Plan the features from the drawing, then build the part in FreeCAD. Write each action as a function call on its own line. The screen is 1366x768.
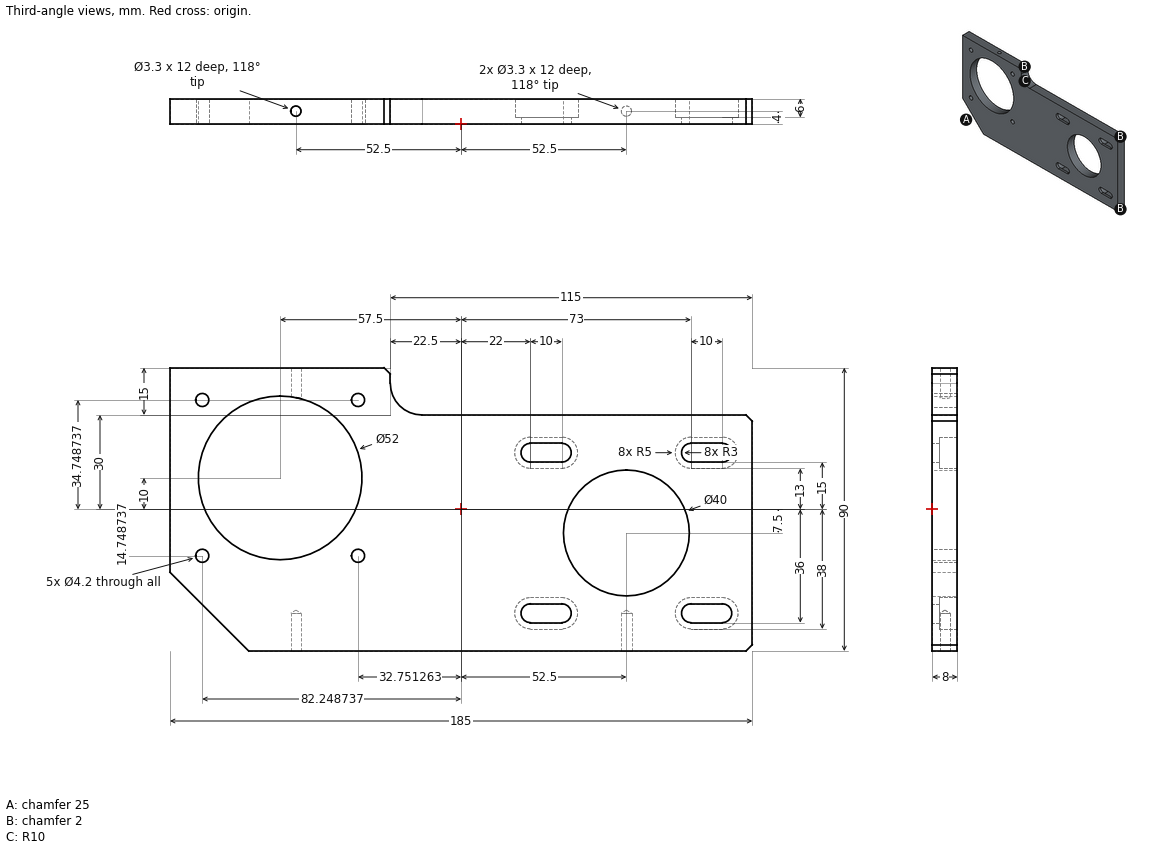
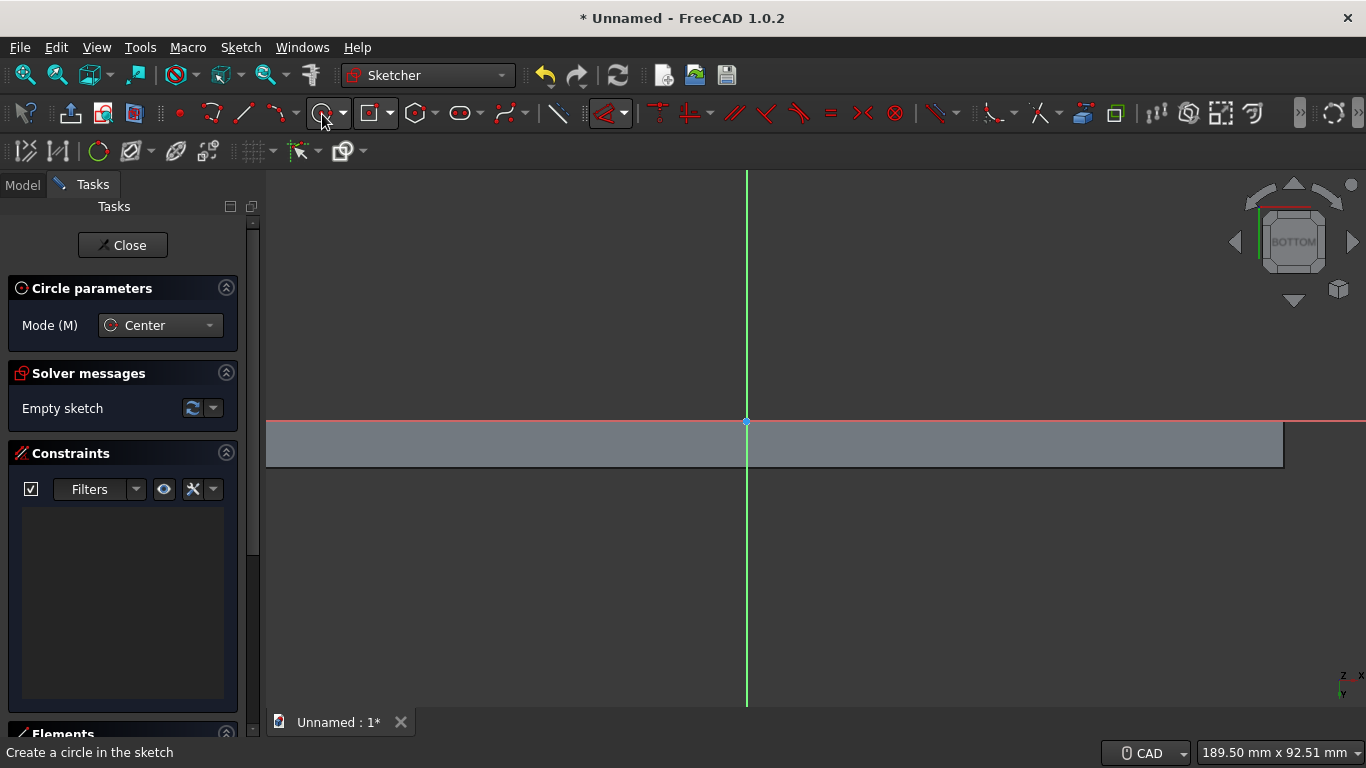
scroll(1051, 445, up, 5)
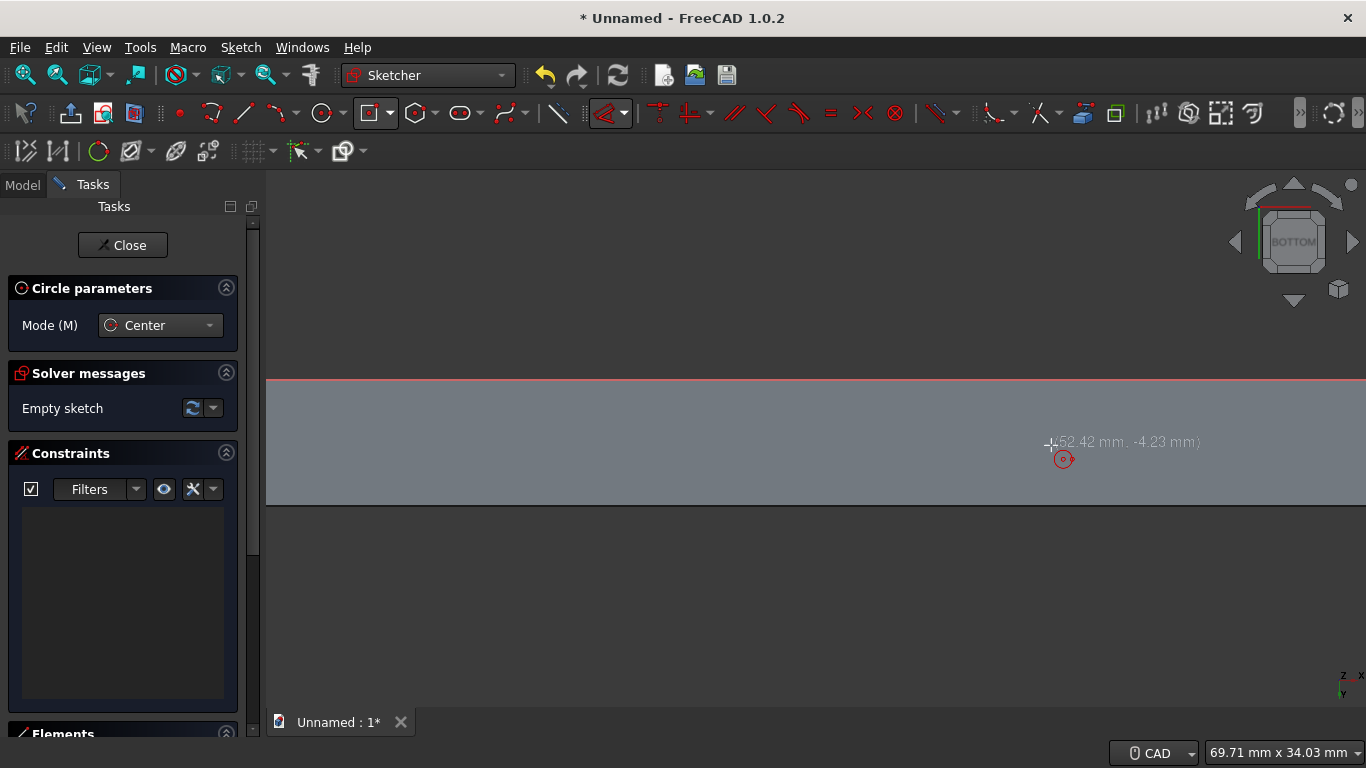
click(1051, 443)
click(1069, 425)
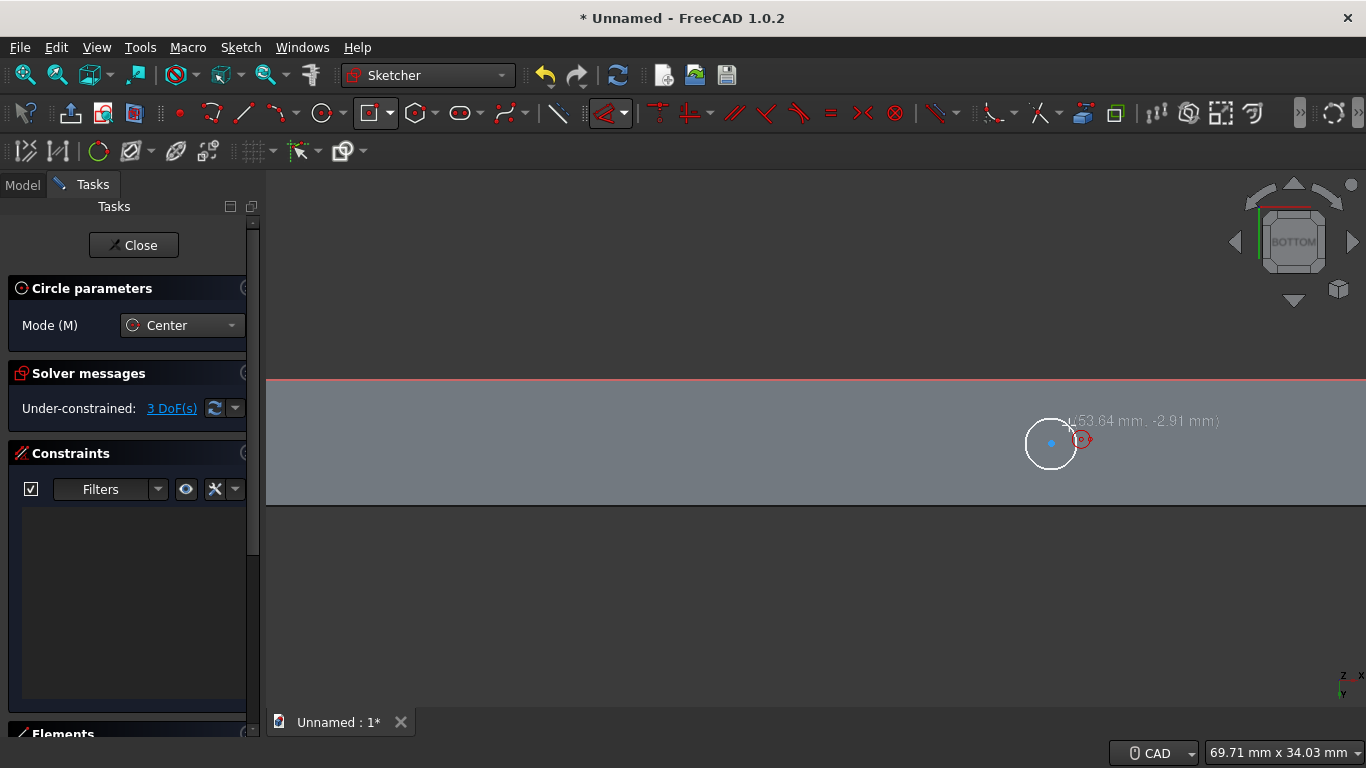
scroll(1053, 447, down, 5)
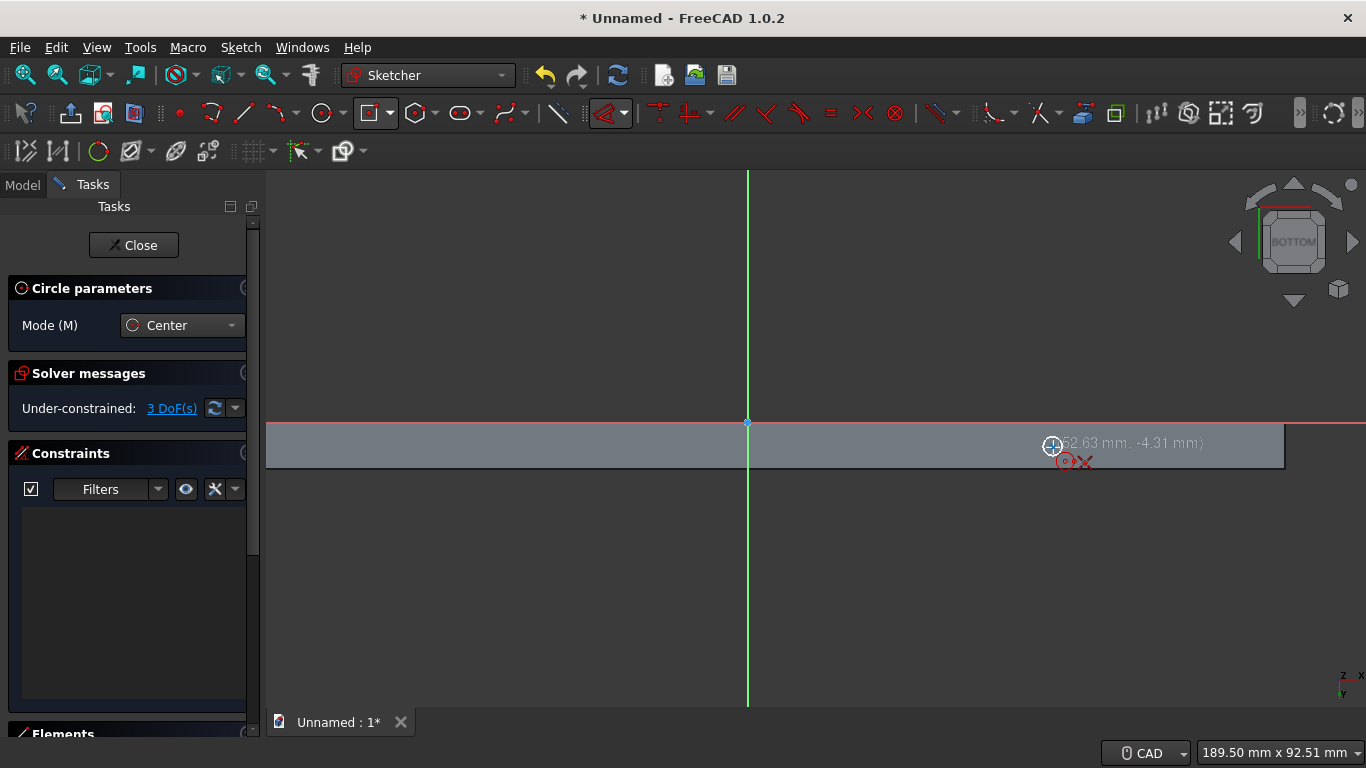
scroll(443, 446, up, 5)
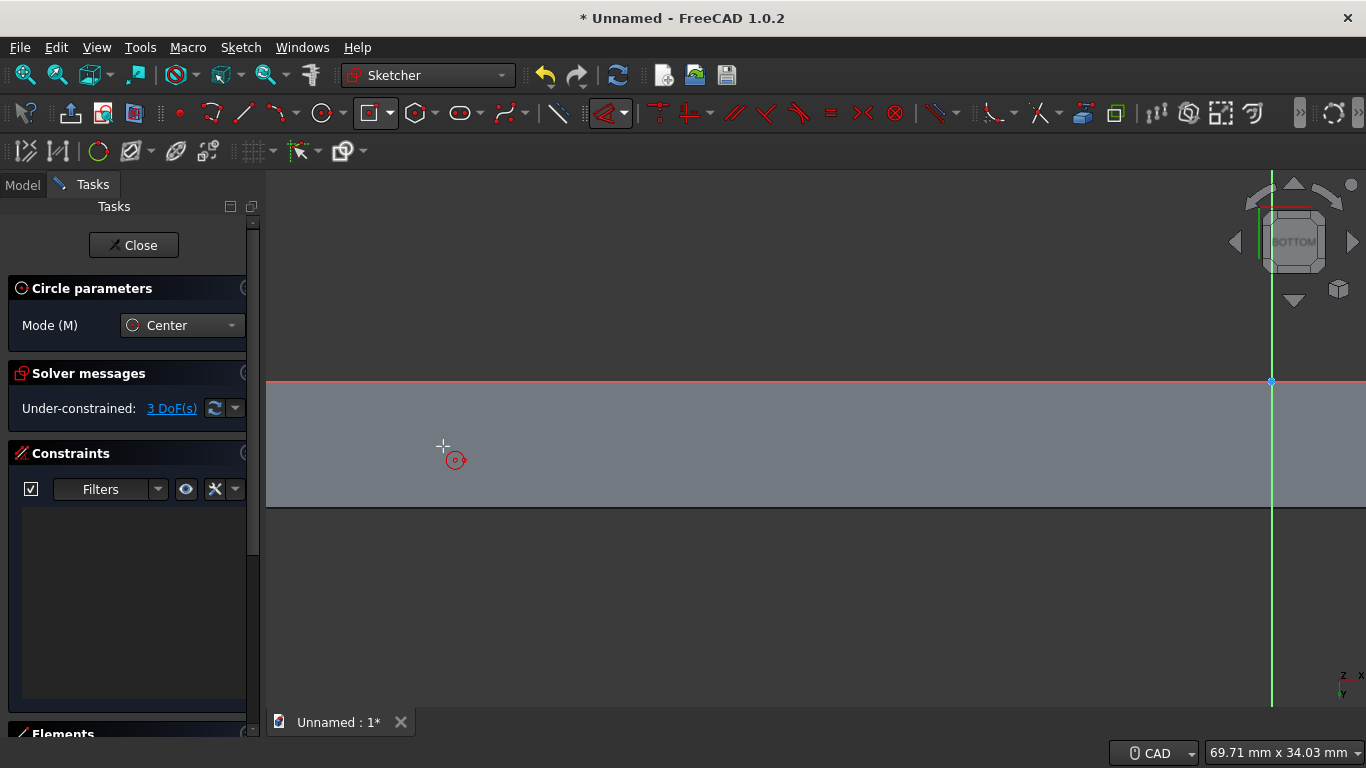
click(443, 445)
click(462, 426)
key(Escape)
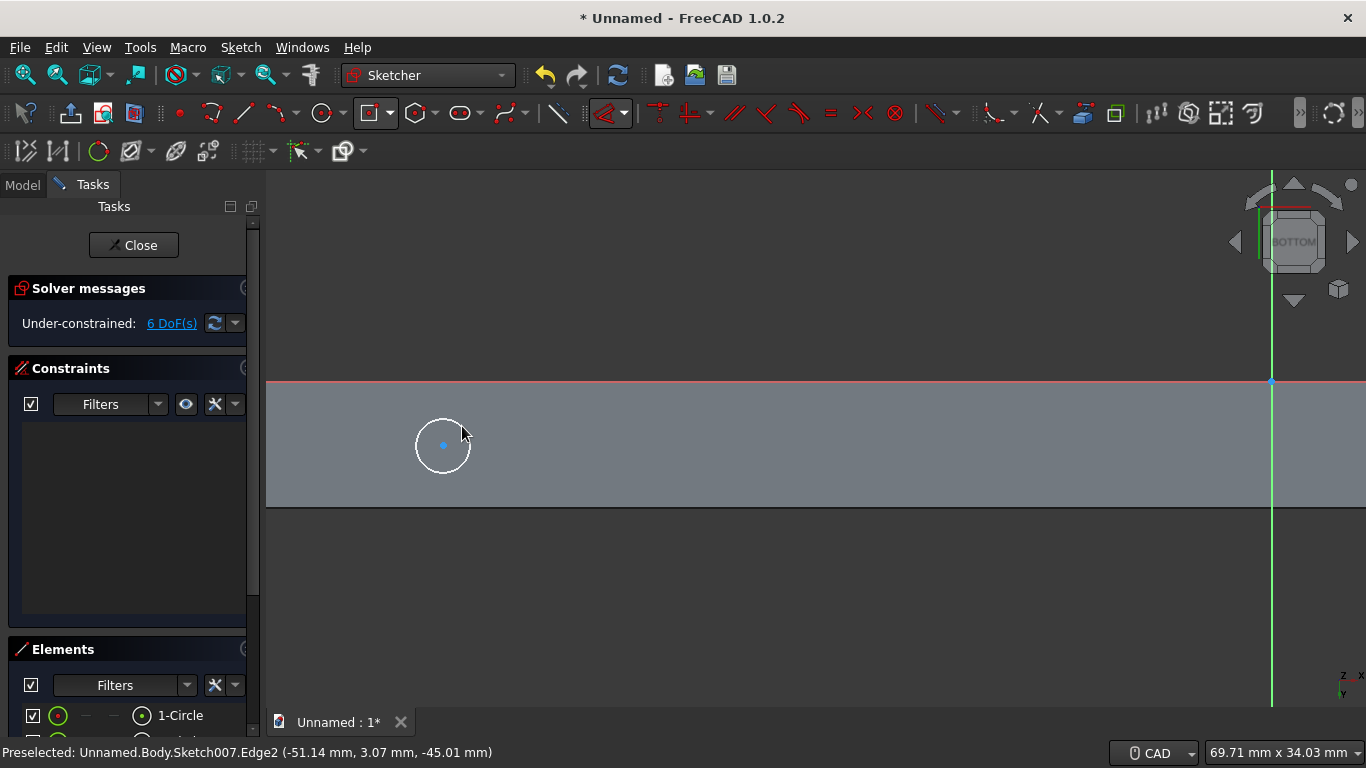
scroll(442, 446, down, 5)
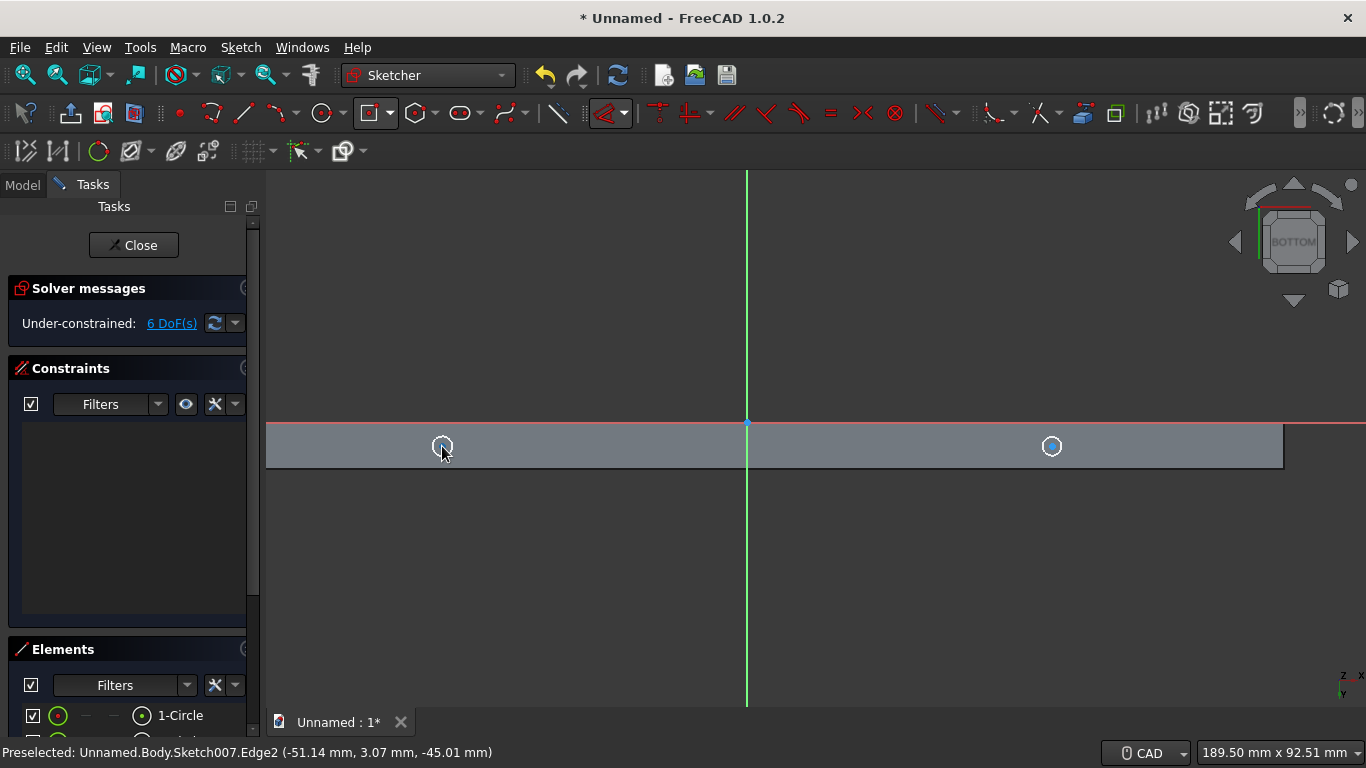
scroll(1059, 440, up, 2)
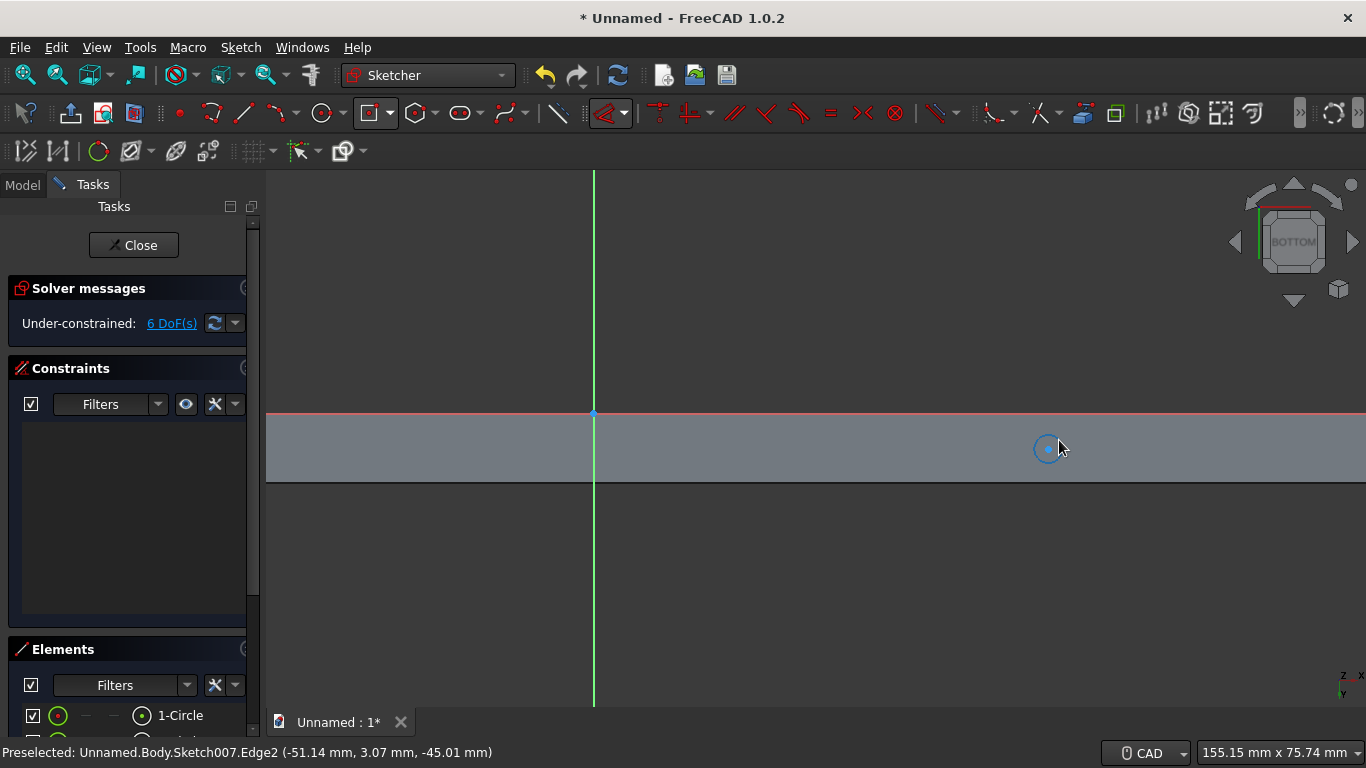
click(1058, 439)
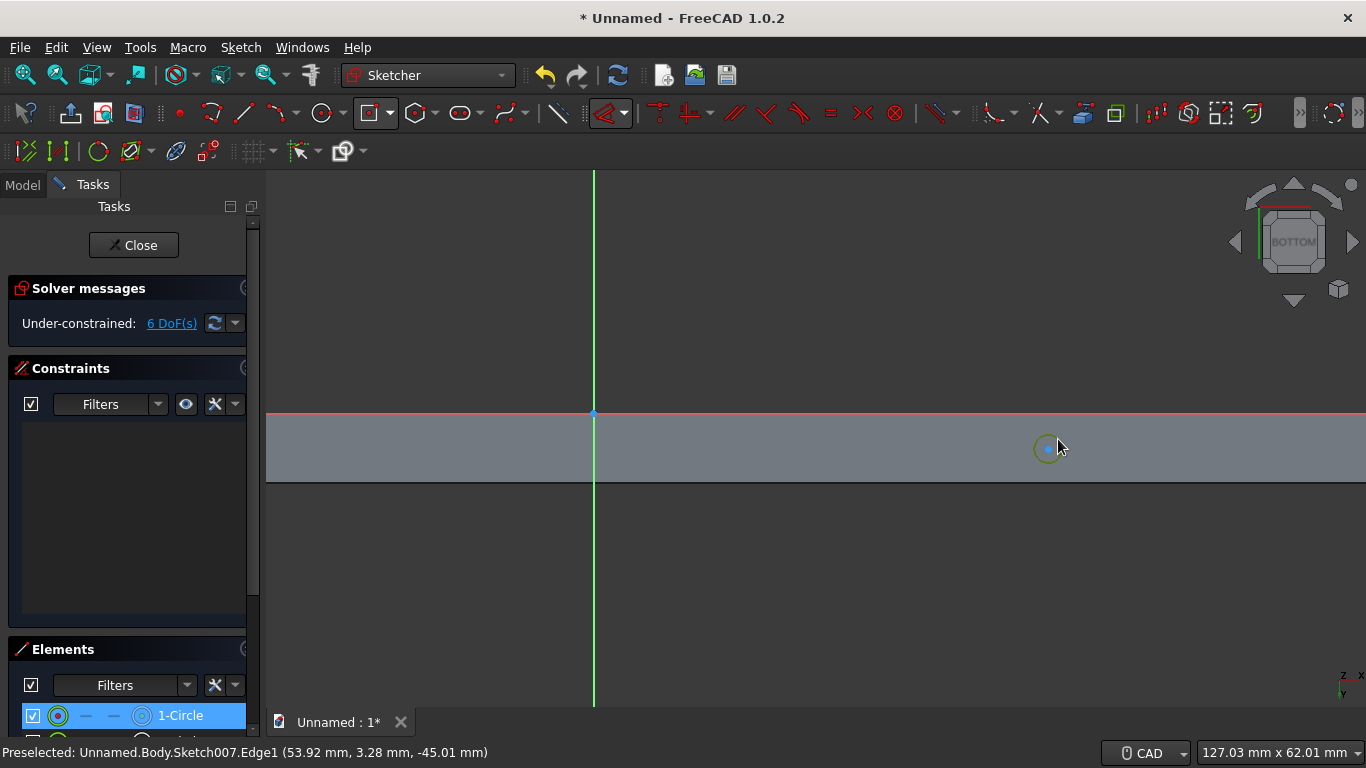
scroll(1060, 439, down, 2)